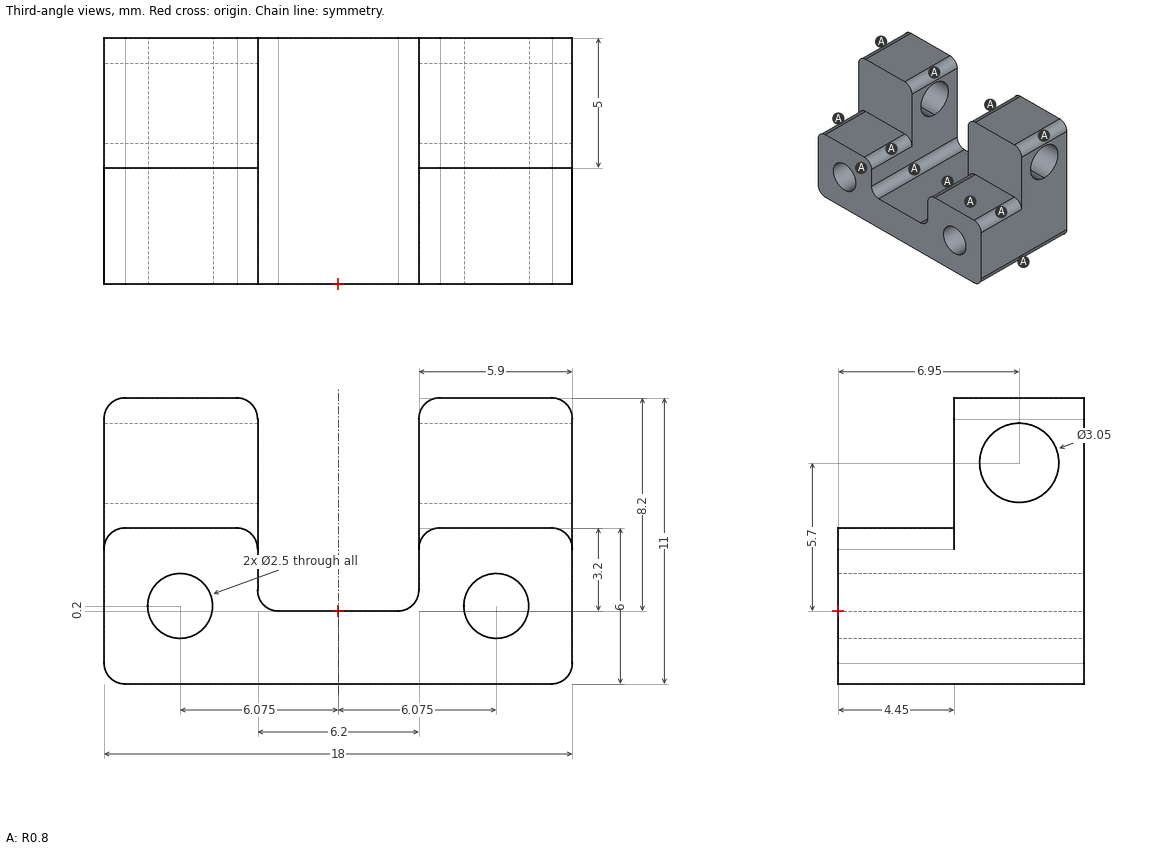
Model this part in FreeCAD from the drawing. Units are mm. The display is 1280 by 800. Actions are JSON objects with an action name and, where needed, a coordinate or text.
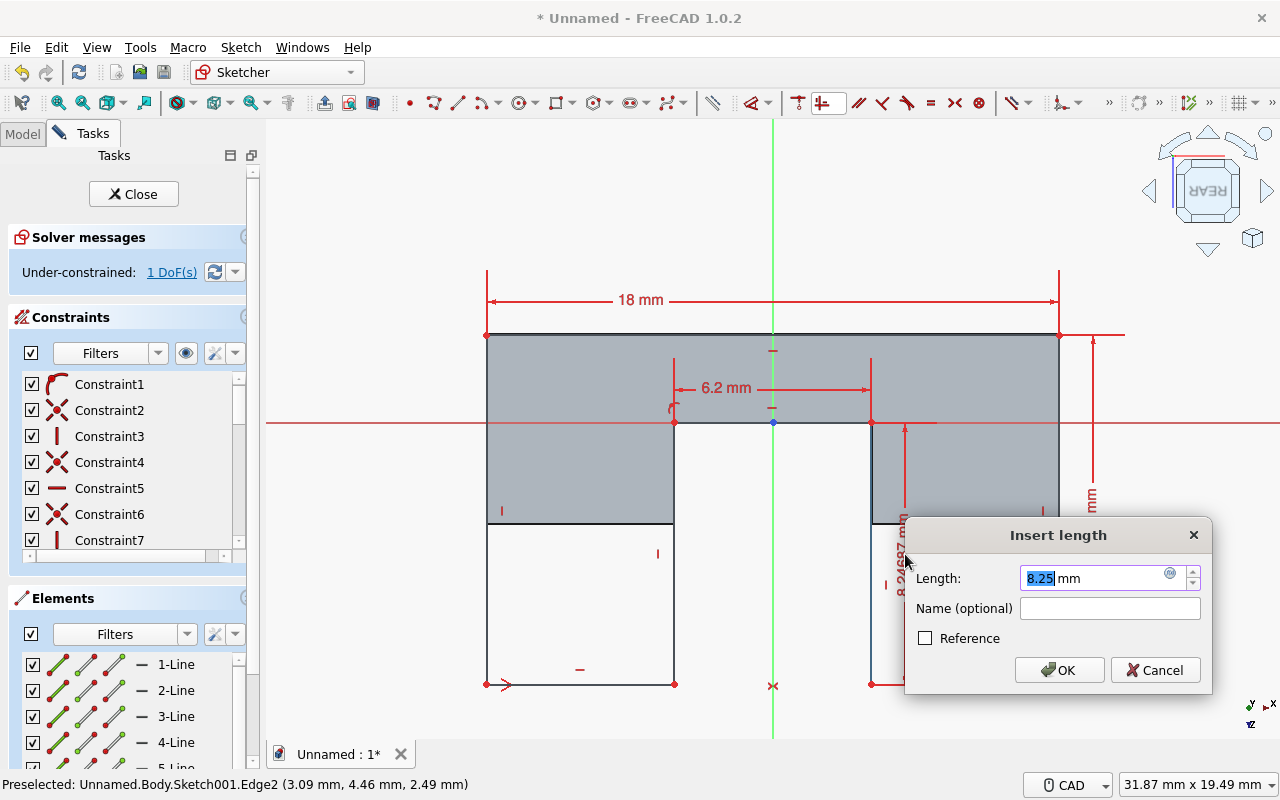
{"action": "type", "text": "8.2"}
{"action": "key", "text": "Return"}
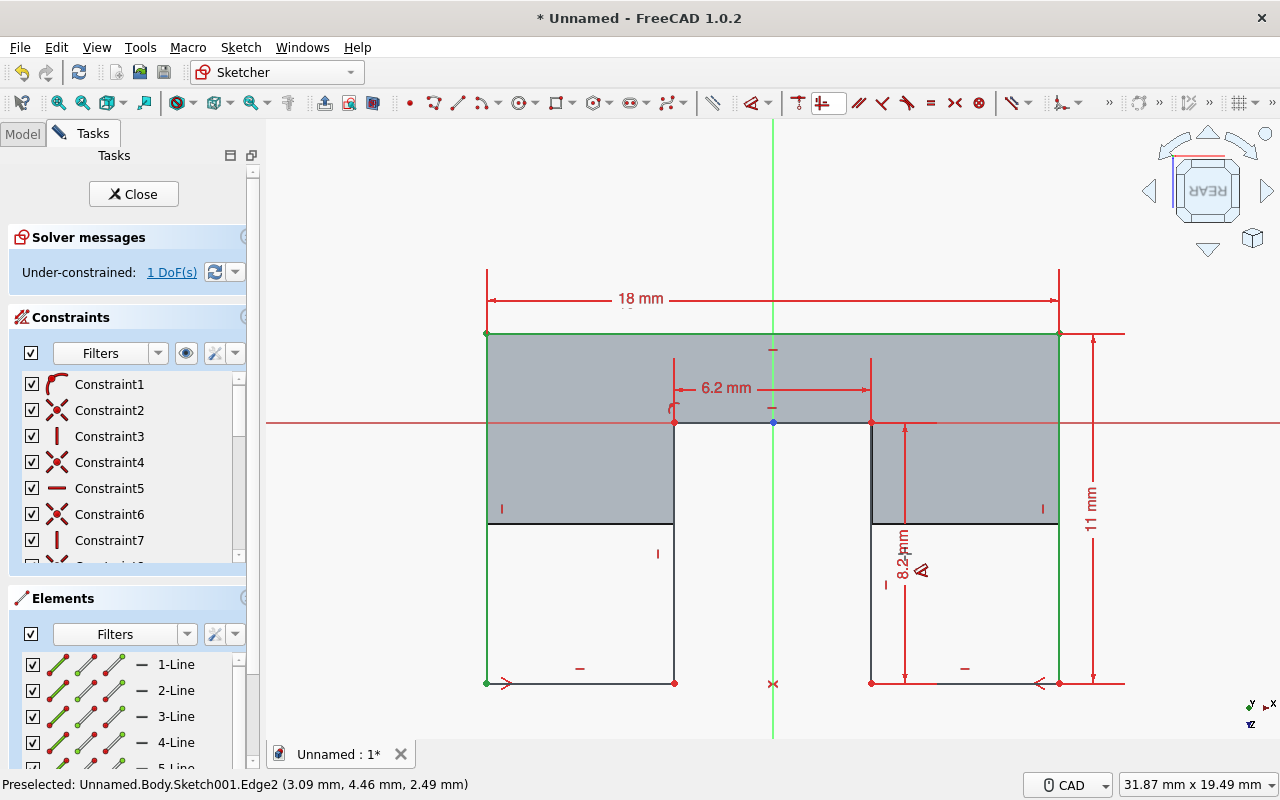
{"action": "left_click", "coordinate": [928, 684]}
{"action": "left_click", "coordinate": [965, 650]}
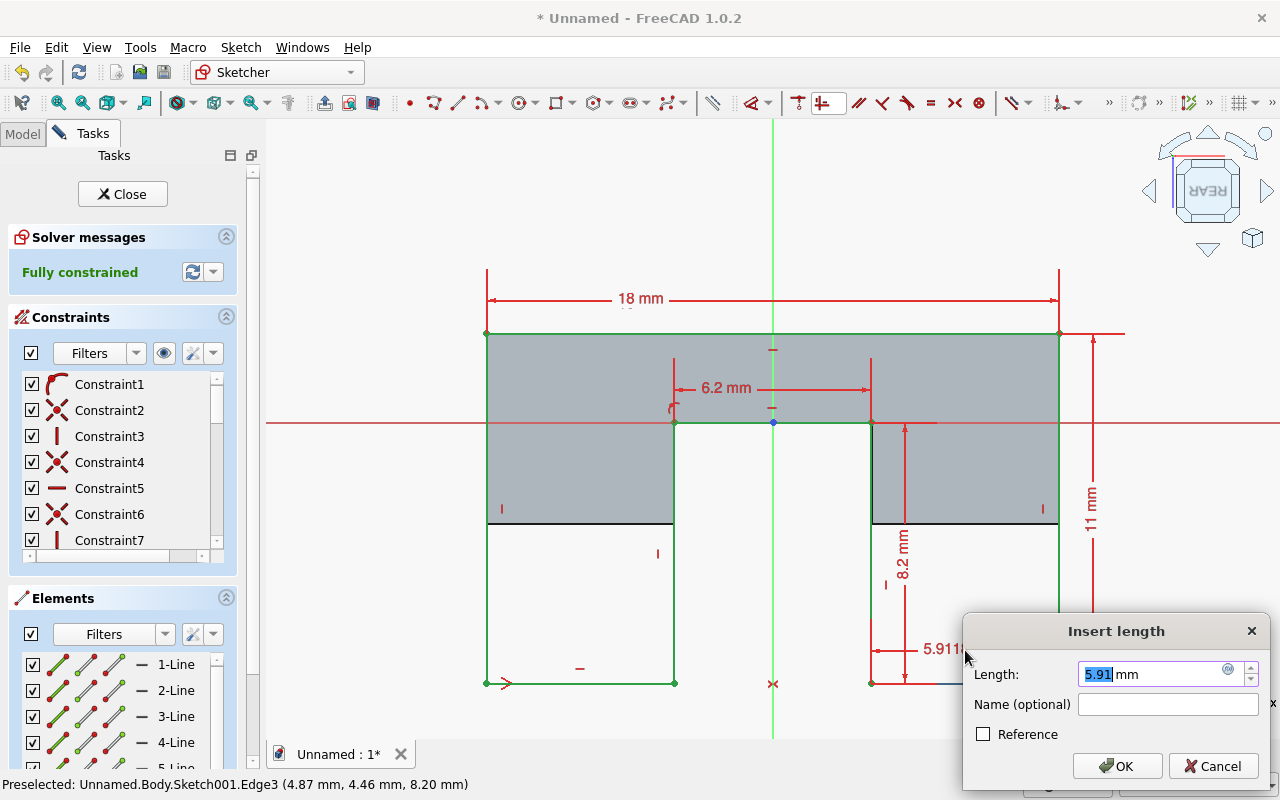
{"action": "type", "text": "5.9"}
{"action": "key", "text": "Return"}
{"action": "key", "text": "Escape"}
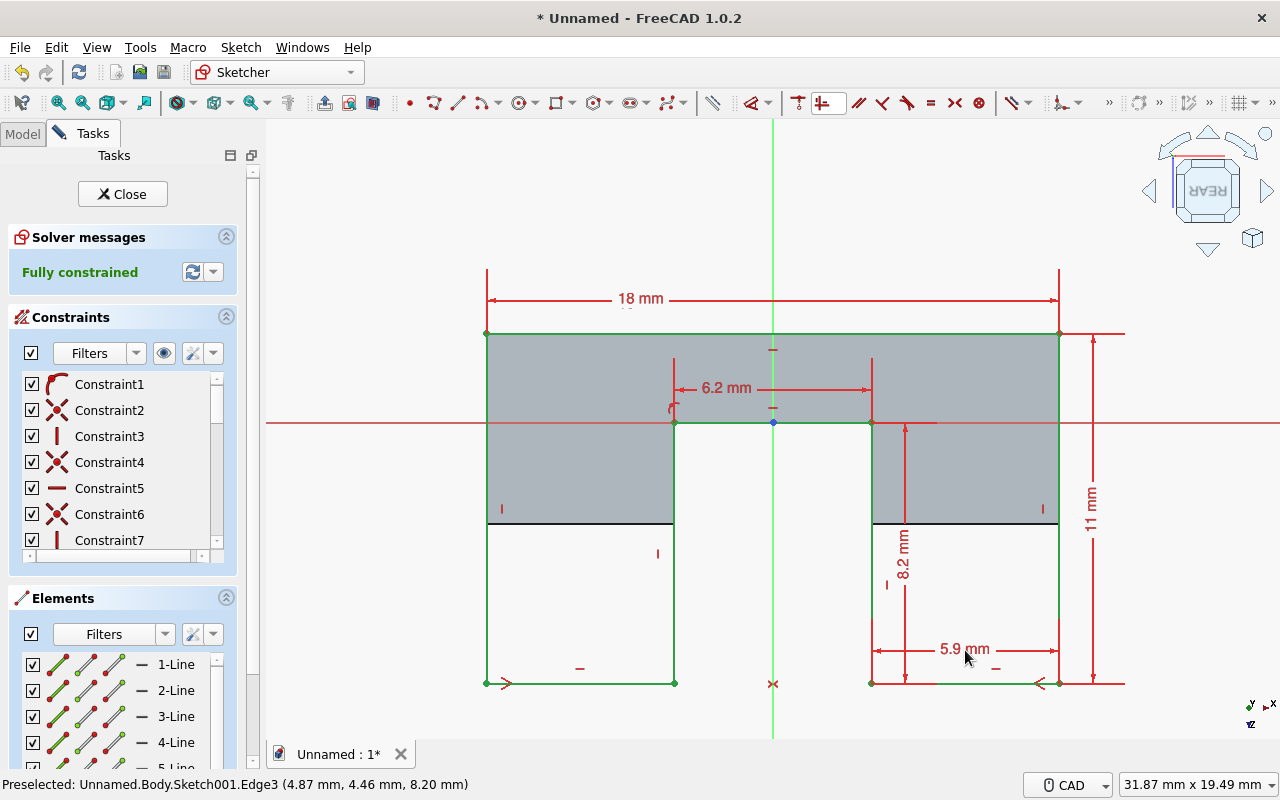
{"action": "left_click", "coordinate": [123, 194]}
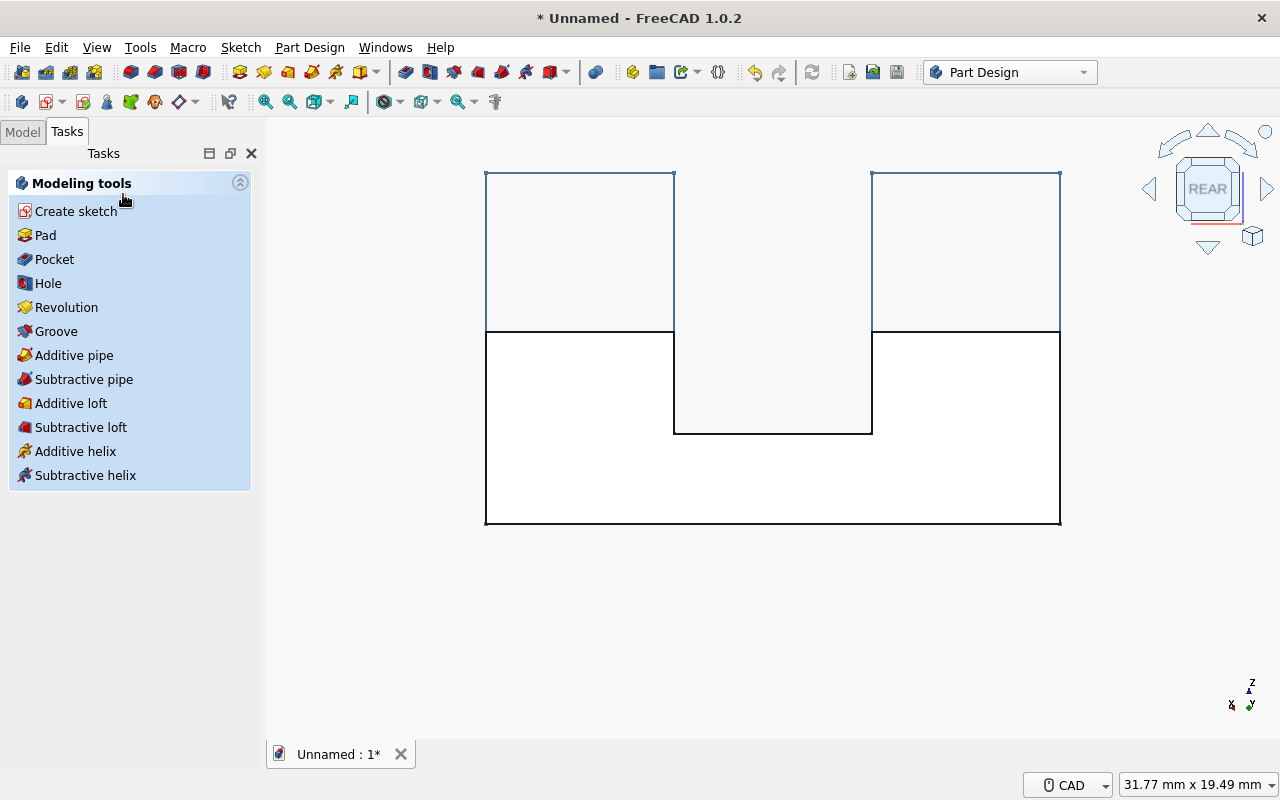
{"action": "left_click", "coordinate": [240, 72]}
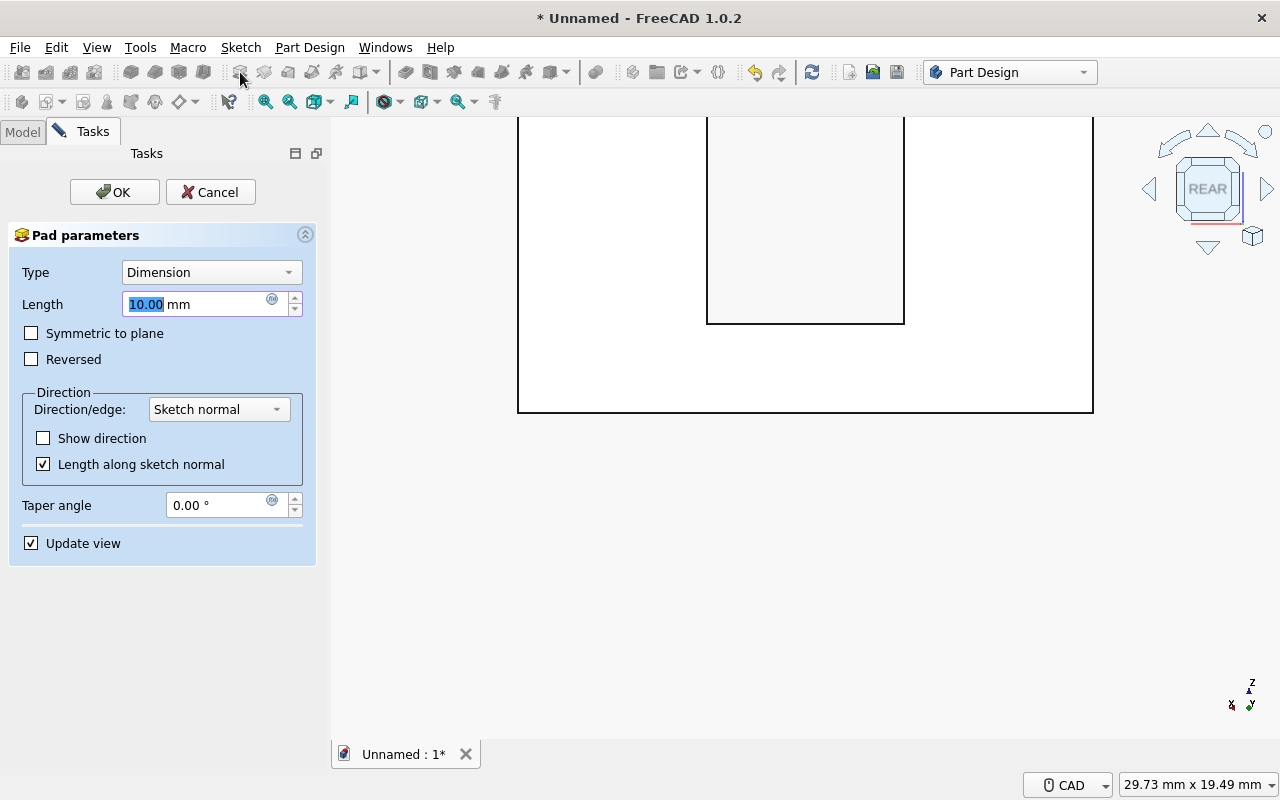
{"action": "type", "text": "5"}
{"action": "key", "text": "Tab"}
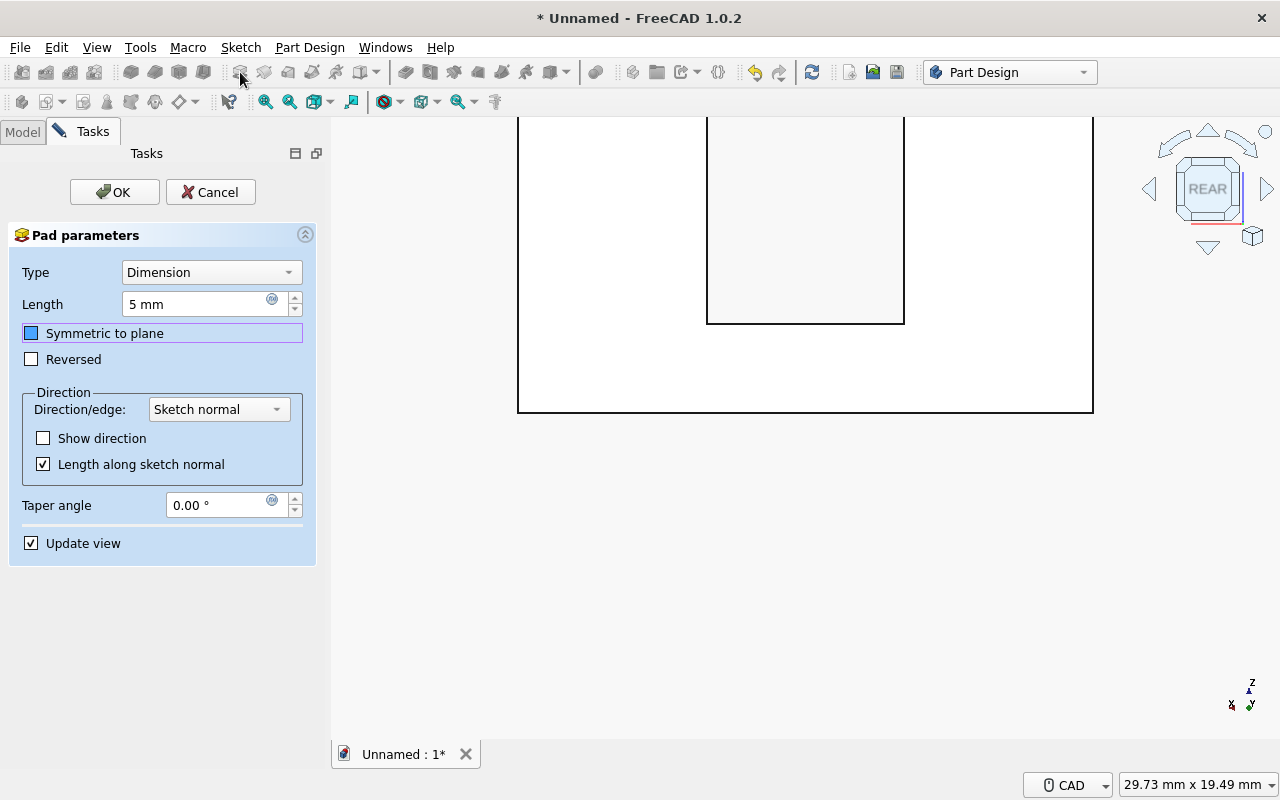
{"action": "left_click", "coordinate": [115, 192]}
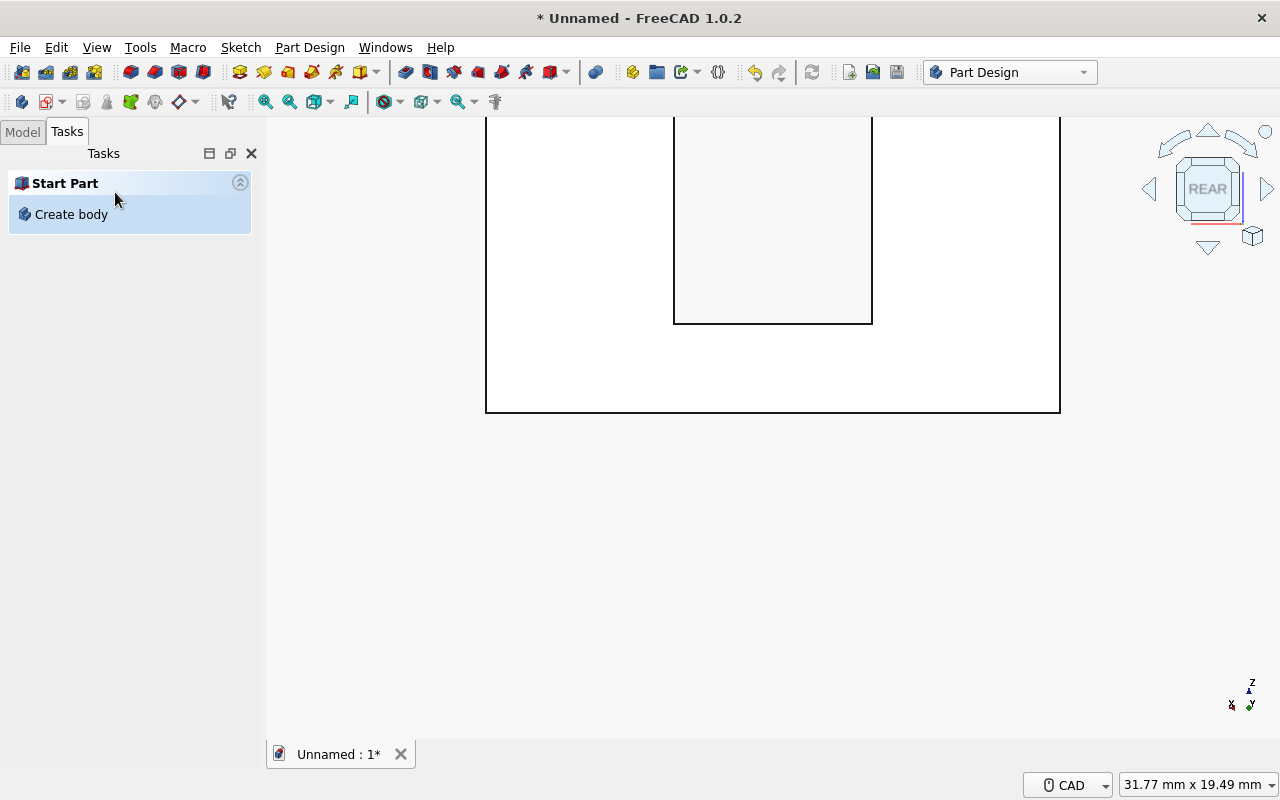
{"action": "left_click", "coordinate": [266, 102]}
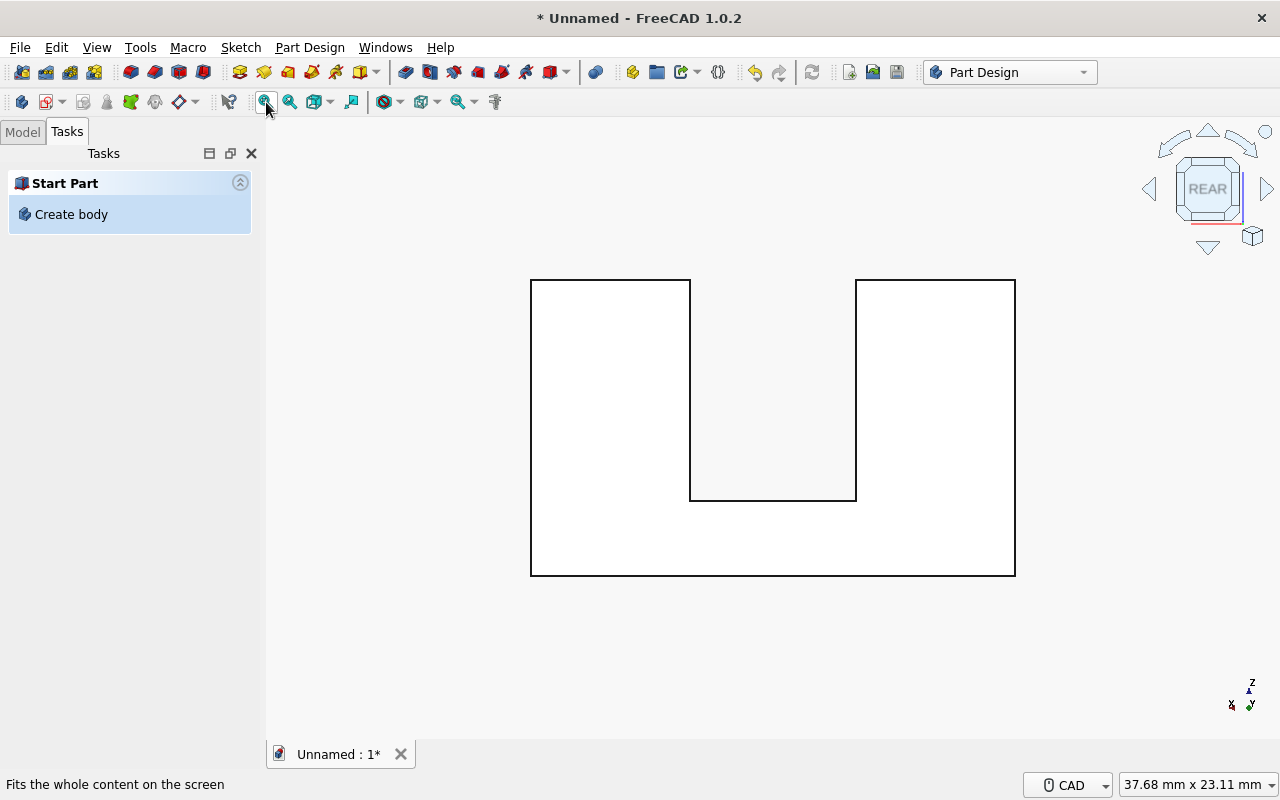
{"action": "left_click", "coordinate": [46, 102]}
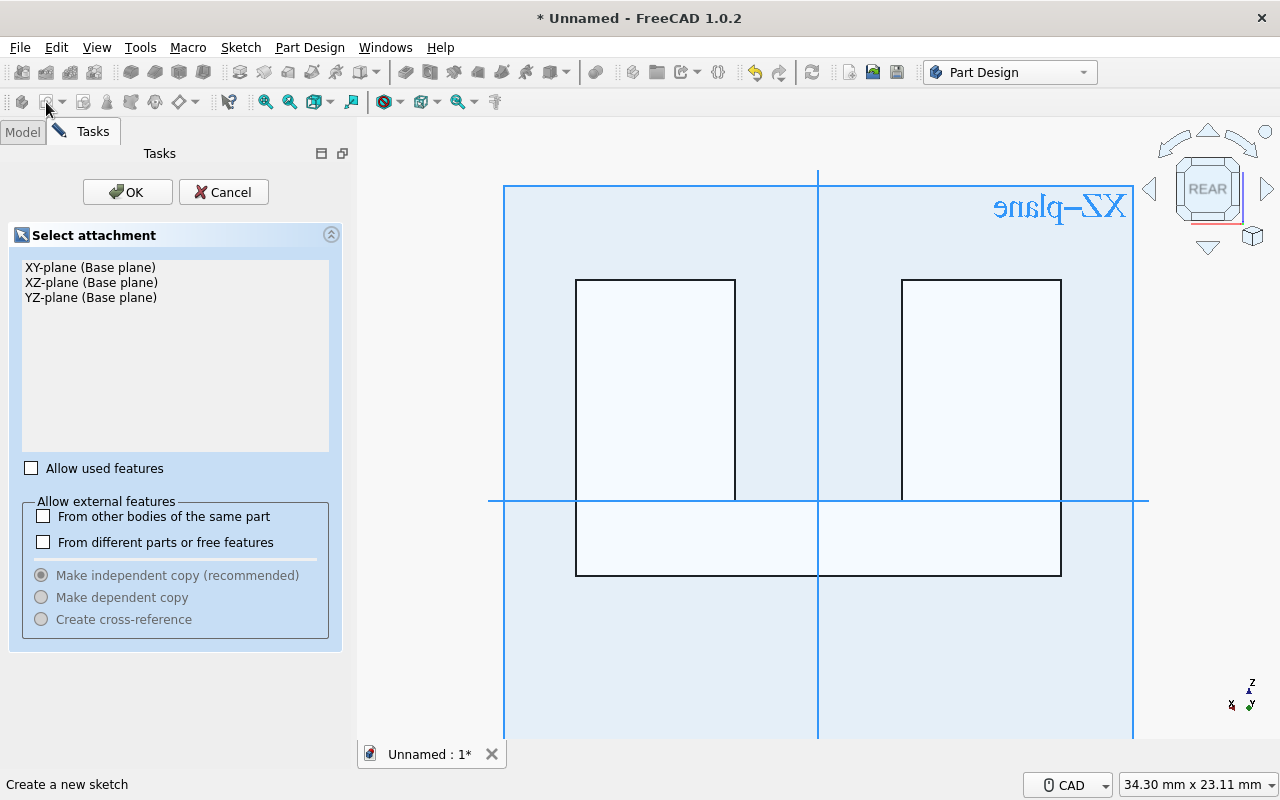
{"action": "left_click", "coordinate": [82, 282]}